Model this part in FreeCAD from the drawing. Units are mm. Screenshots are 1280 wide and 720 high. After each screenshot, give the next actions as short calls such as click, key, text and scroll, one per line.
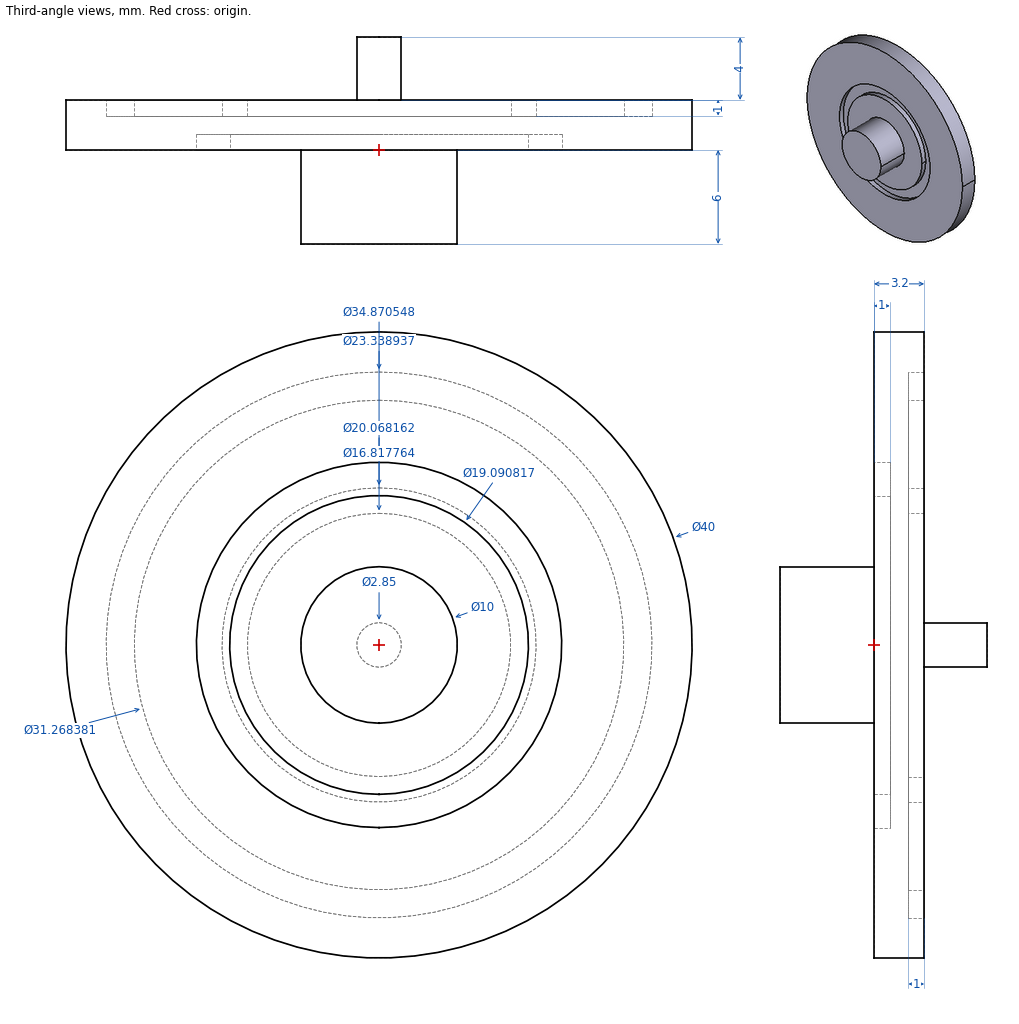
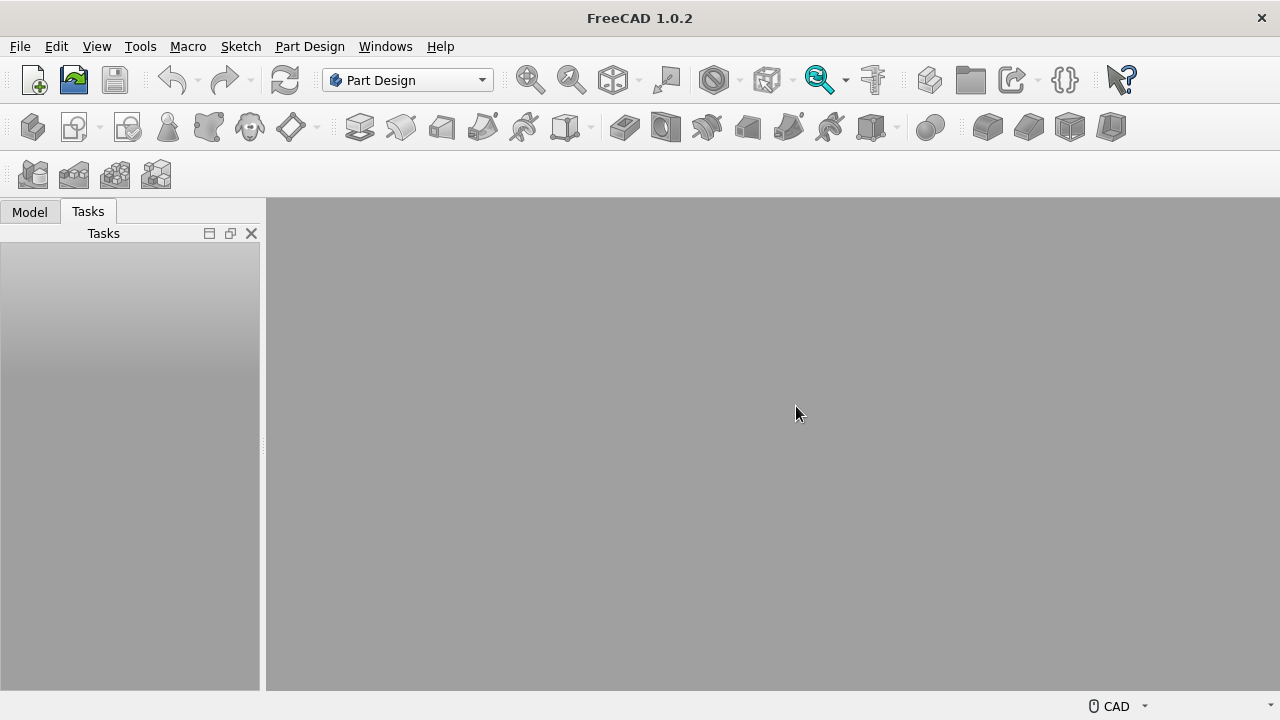
click(33, 80)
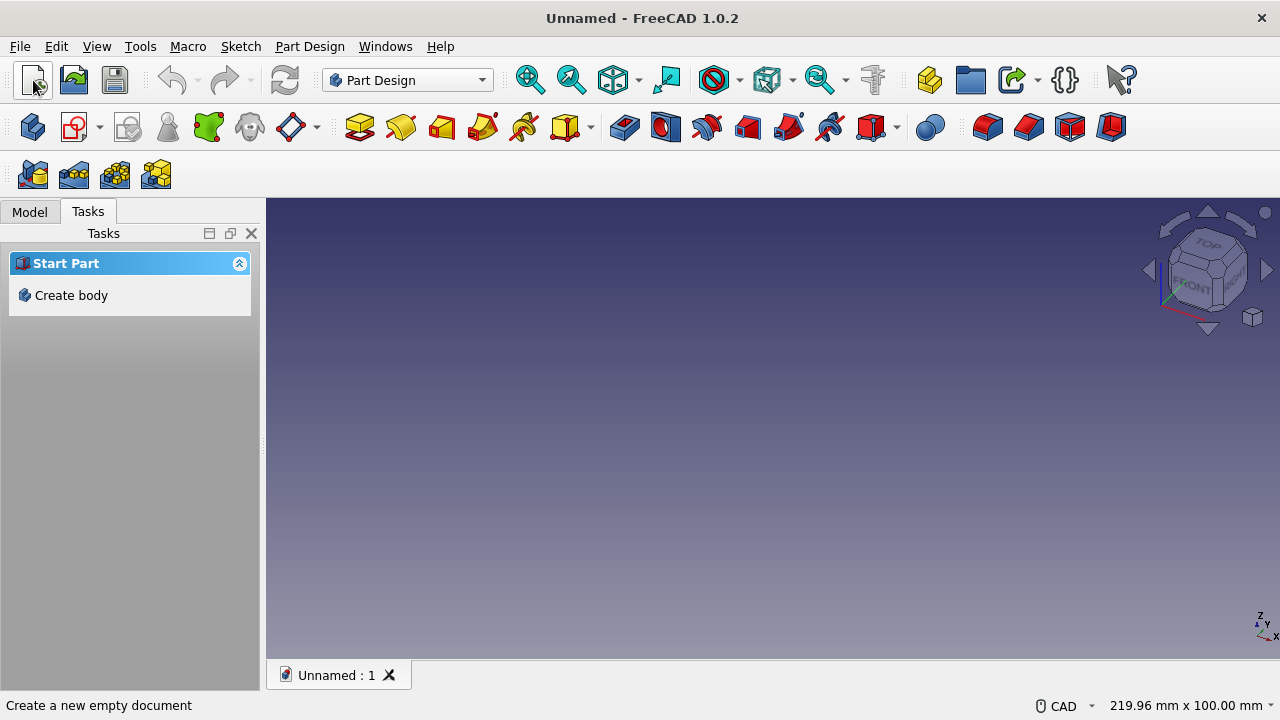
click(74, 128)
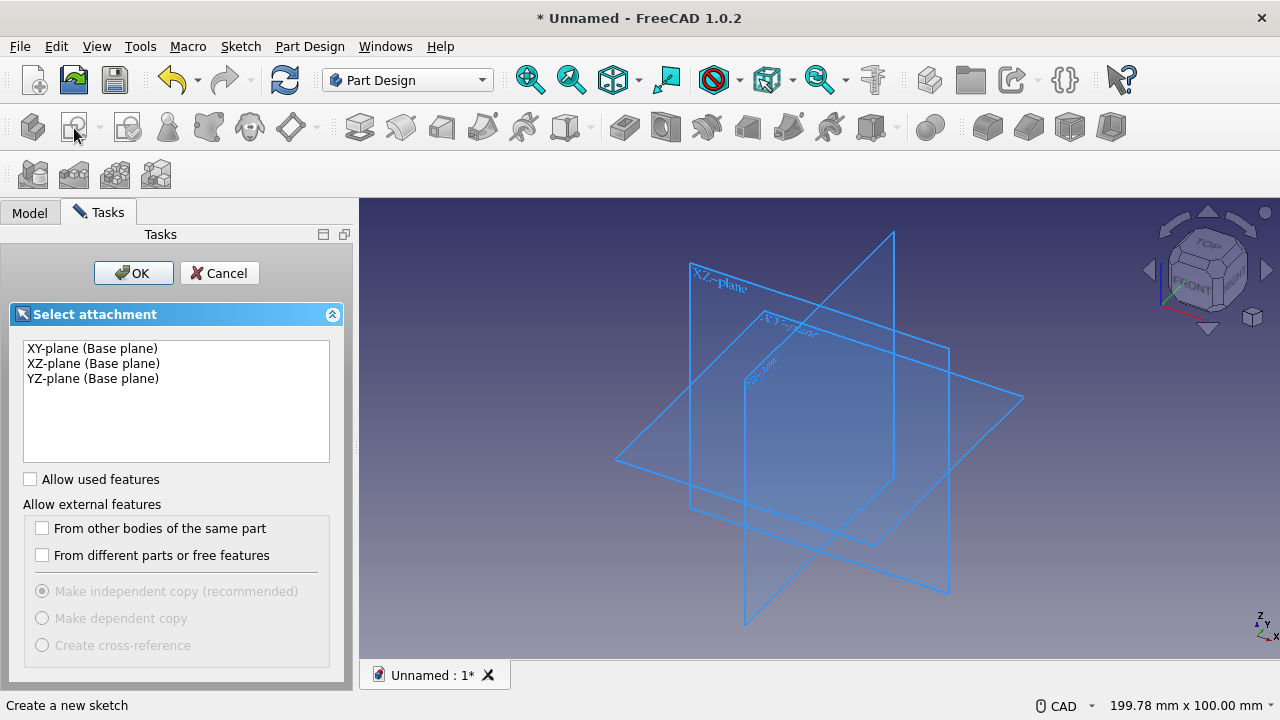
click(84, 364)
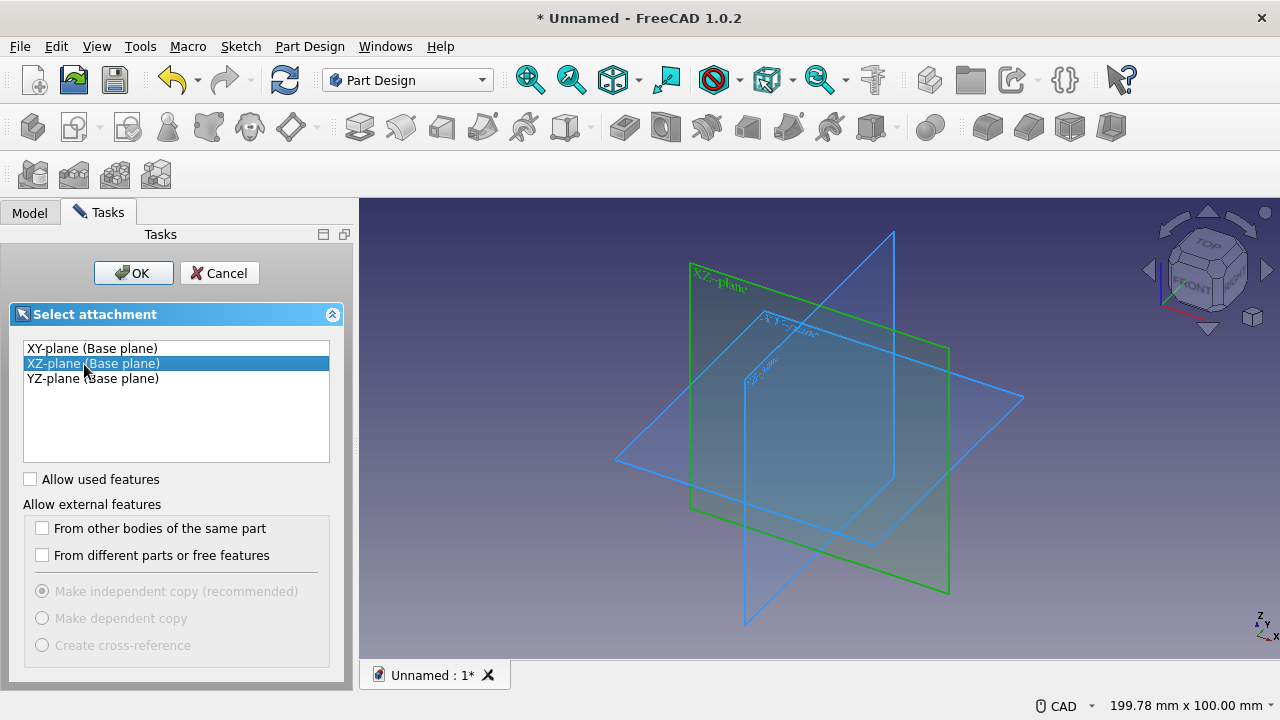
click(134, 273)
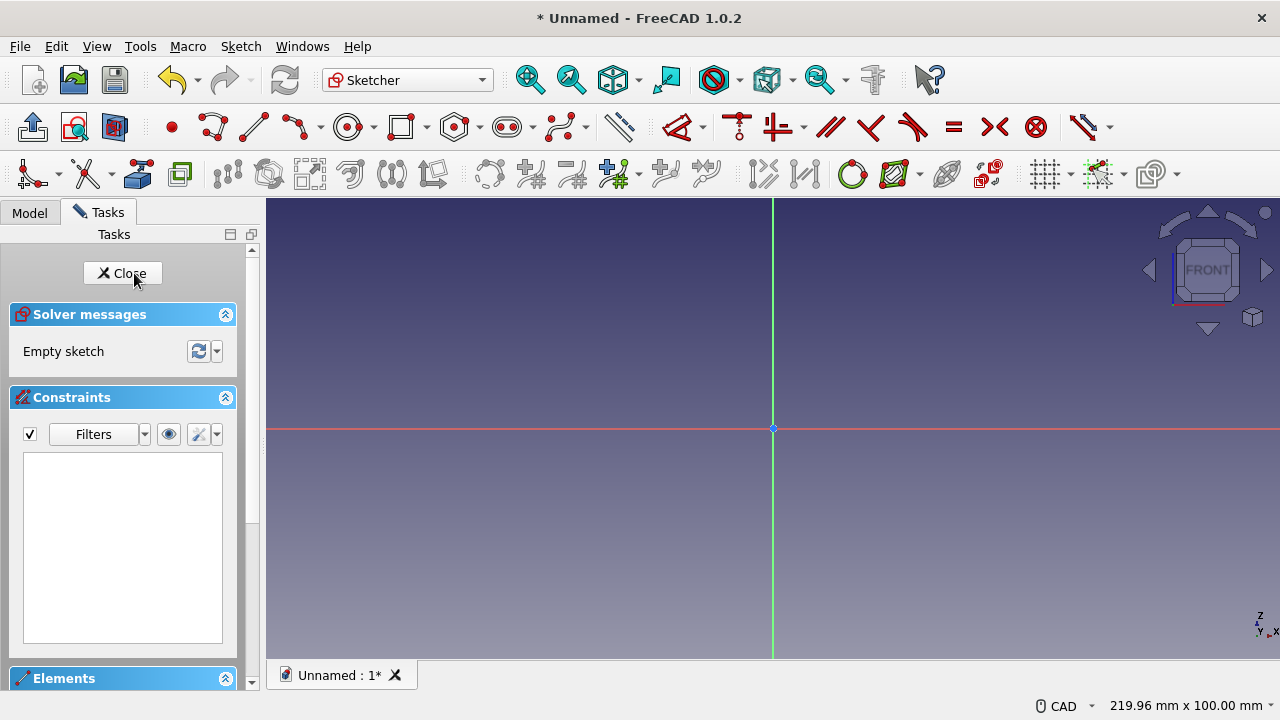
scroll(912, 428, up, 2)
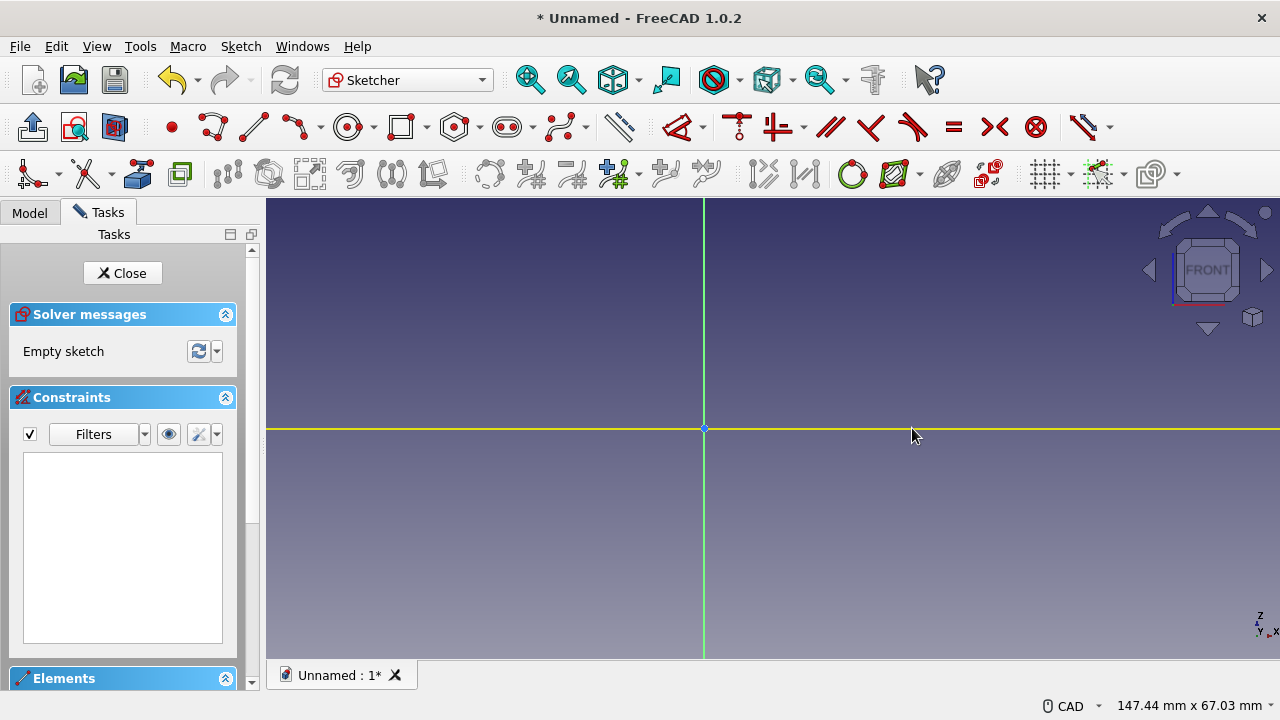
click(348, 128)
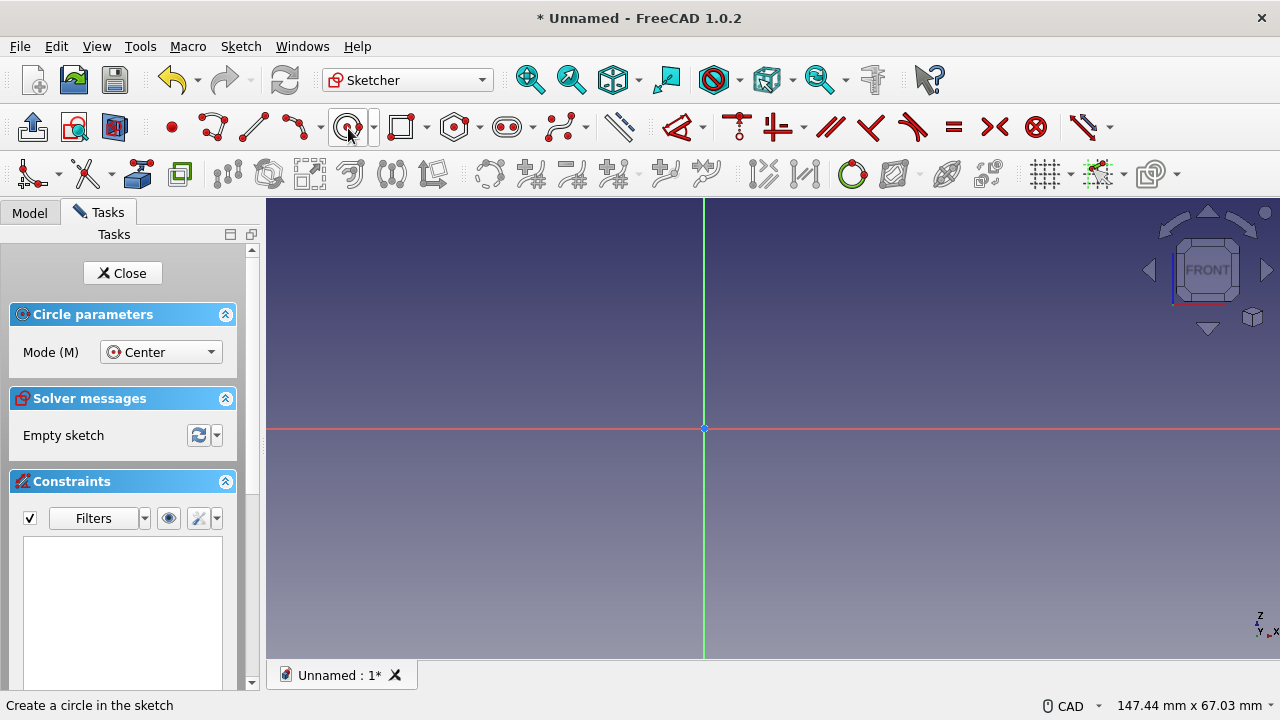
click(704, 428)
move(802, 331)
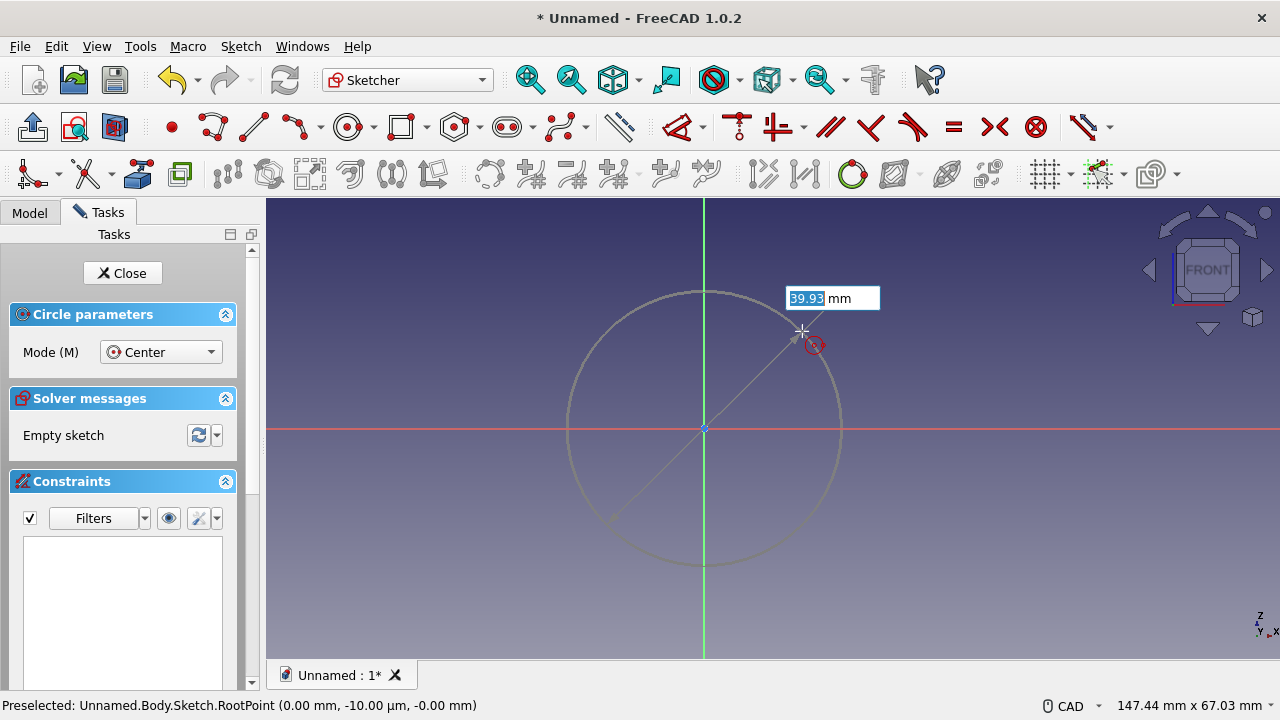
text(40)
key(Return)
key(Escape)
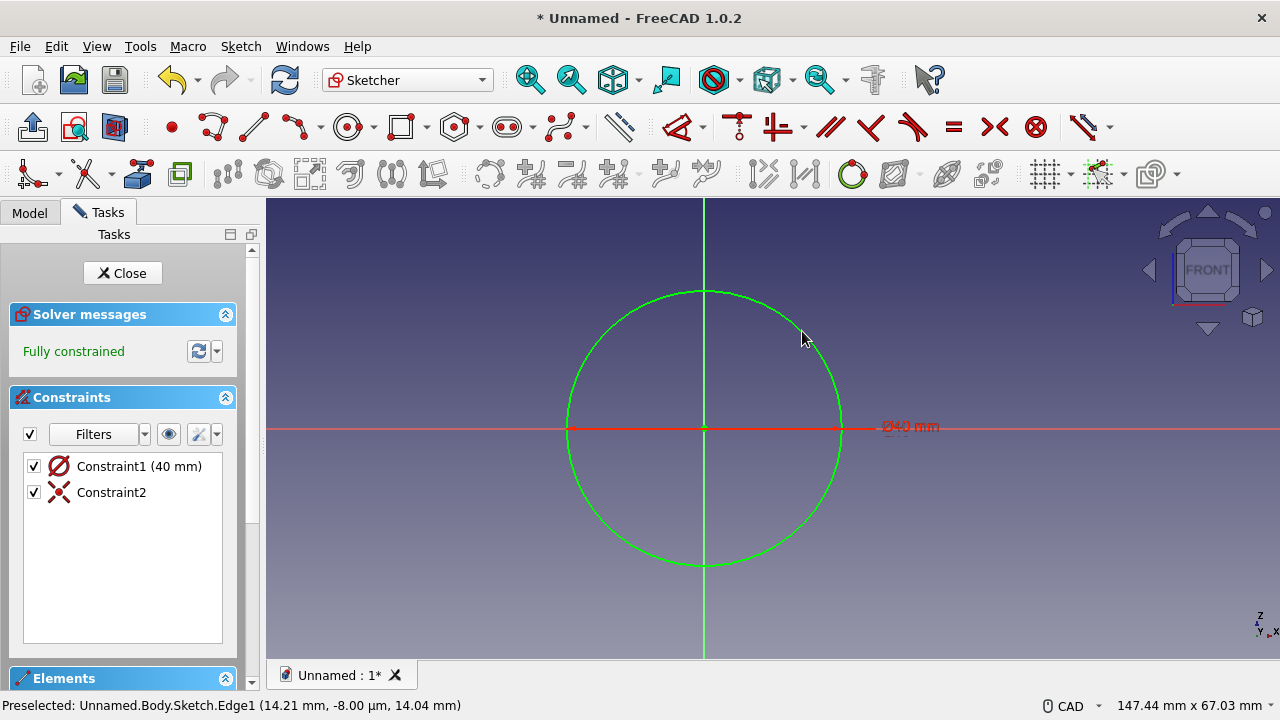
click(123, 273)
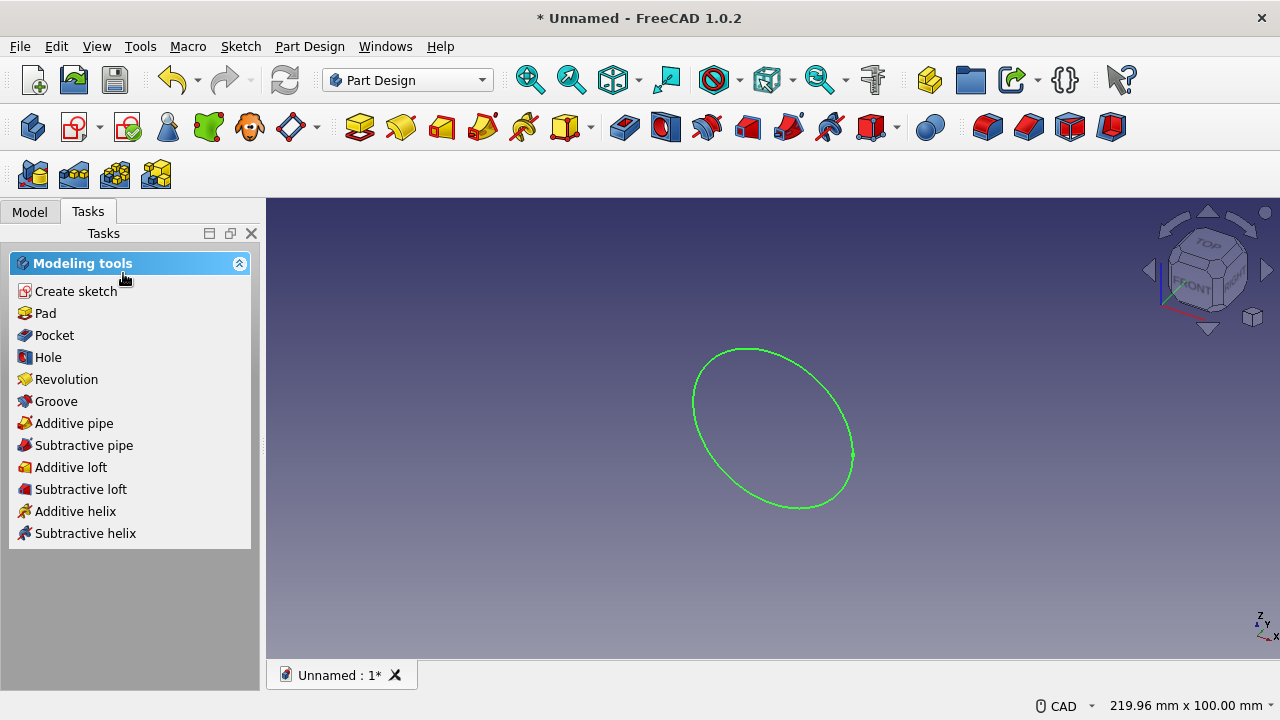
click(360, 128)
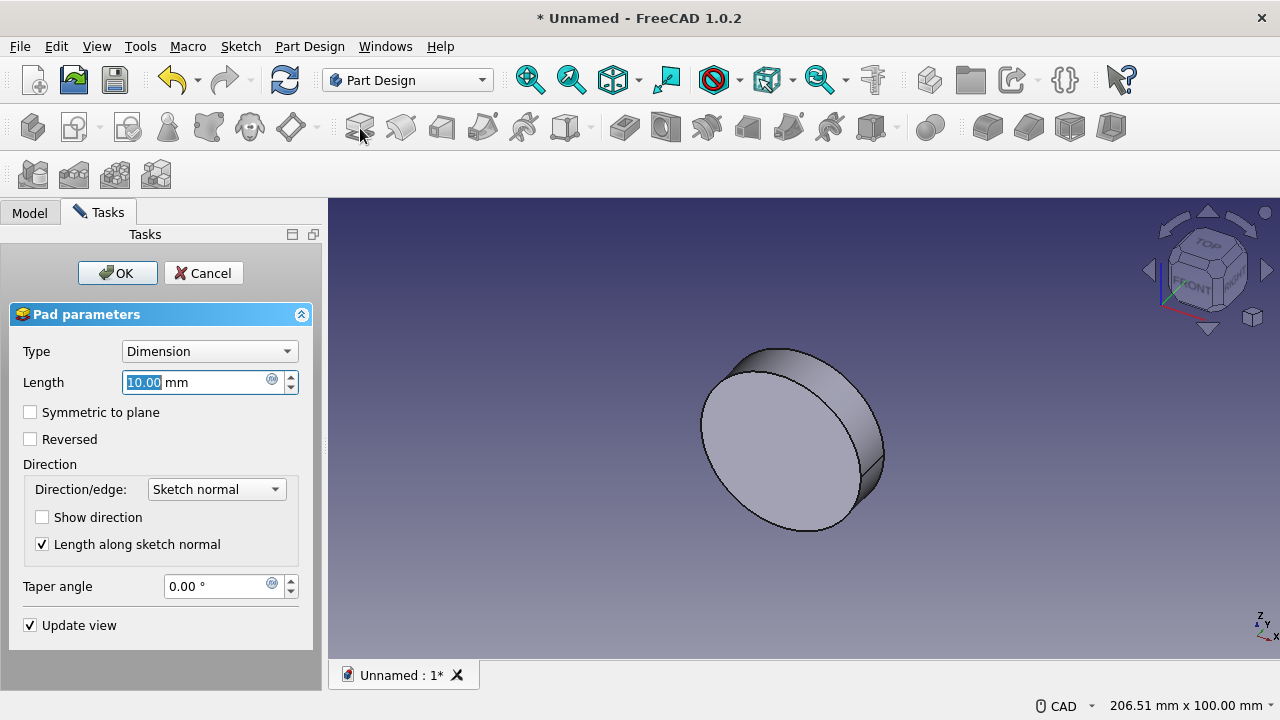
text(3.2)
key(Tab)